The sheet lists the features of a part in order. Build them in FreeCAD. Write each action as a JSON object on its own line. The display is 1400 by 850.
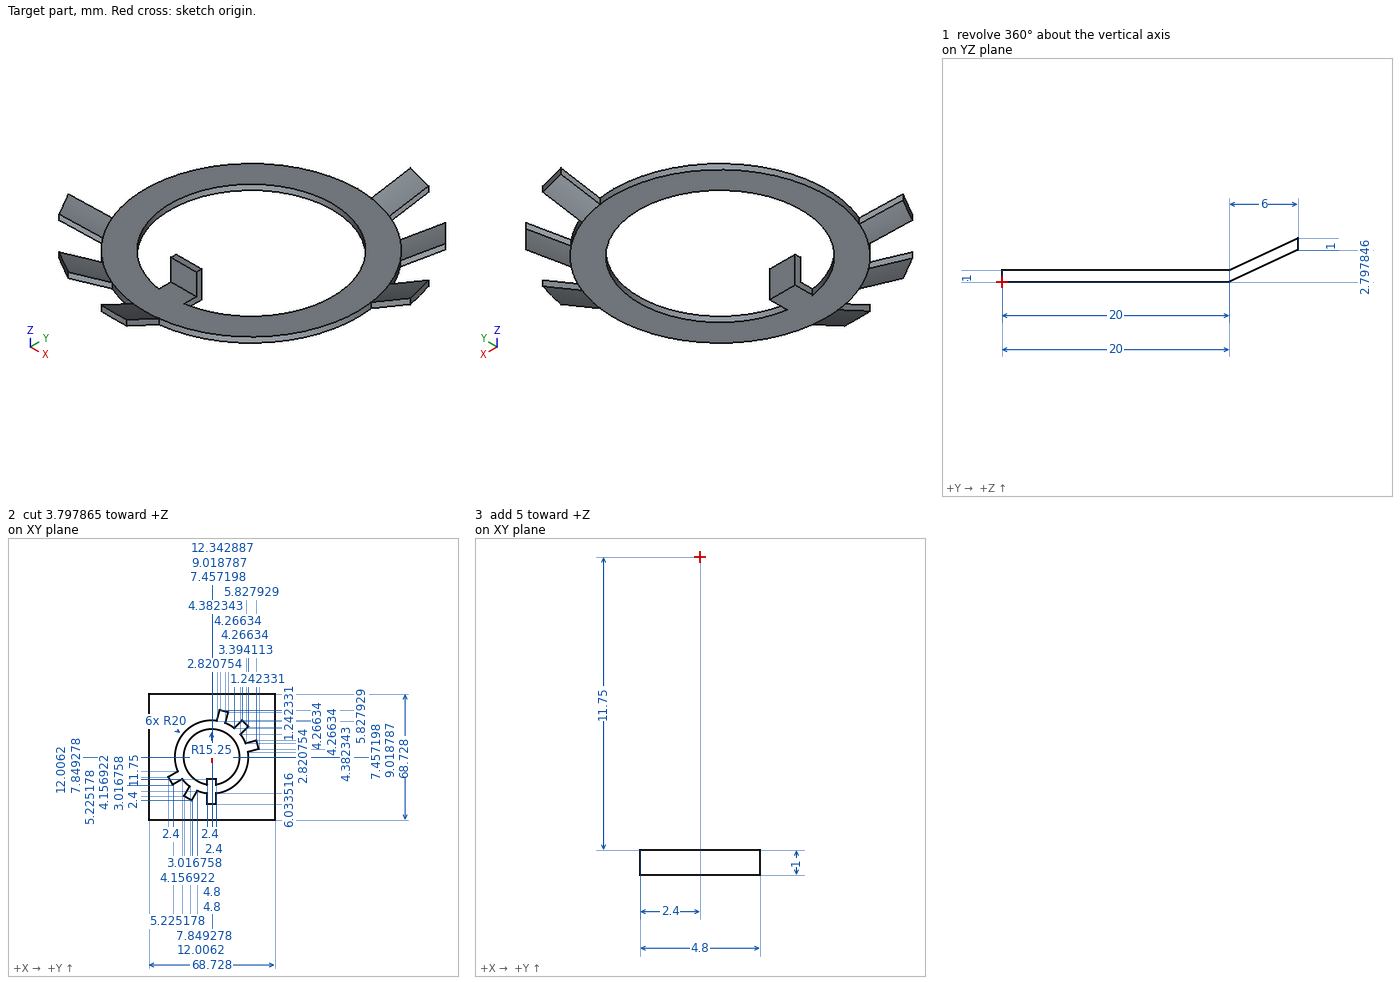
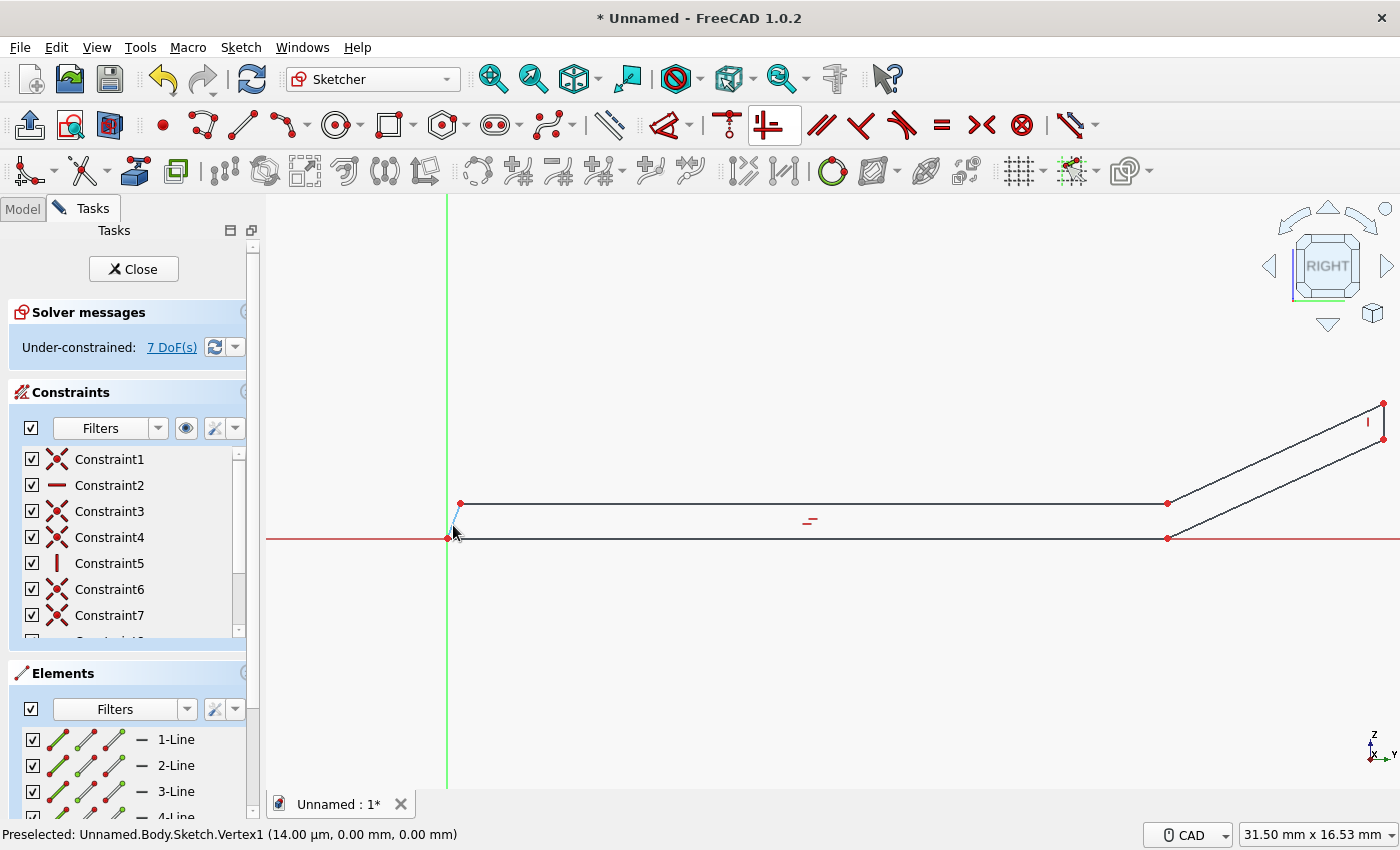
{"action": "left_click", "coordinate": [453, 525]}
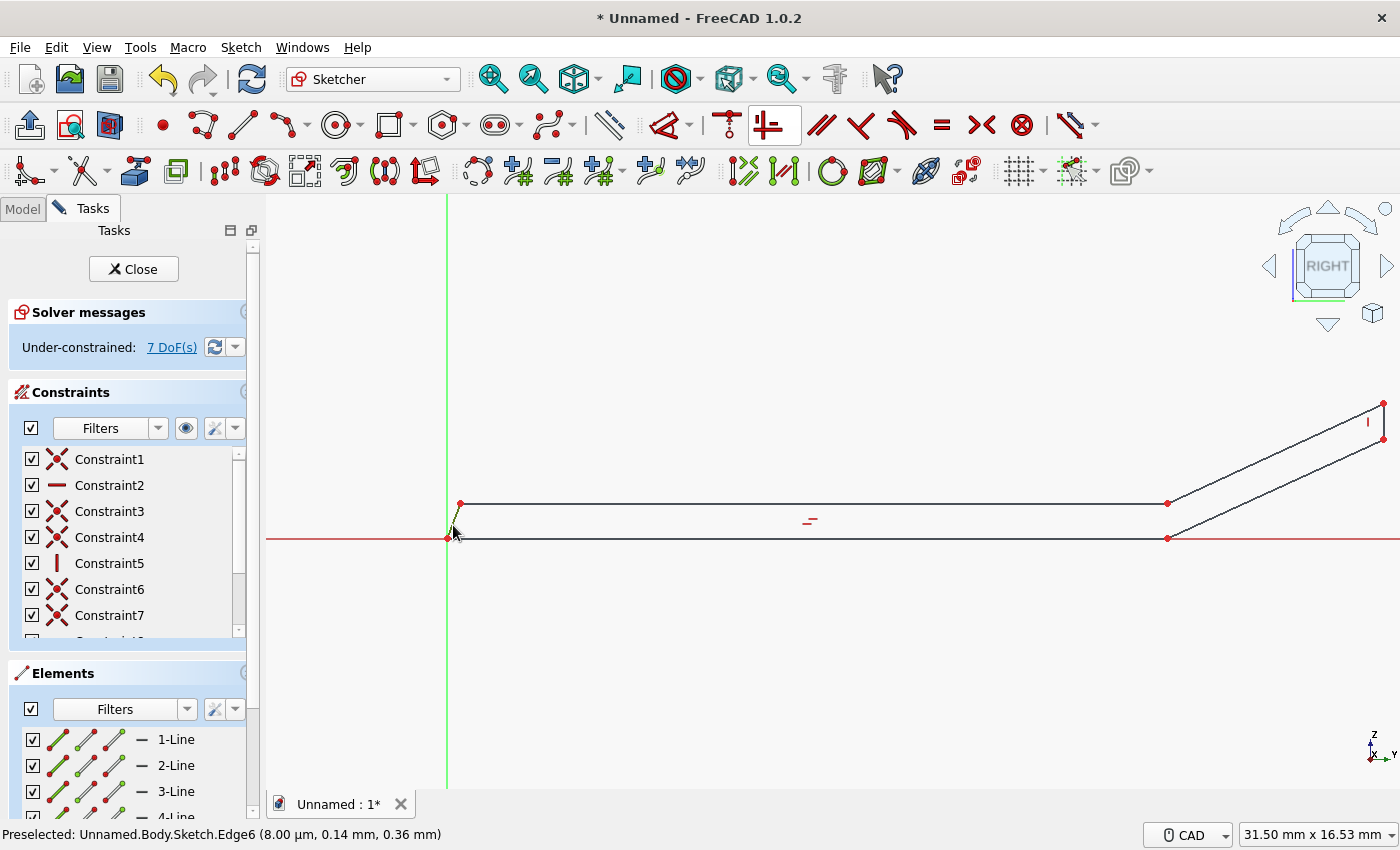
{"action": "left_click", "coordinate": [796, 126]}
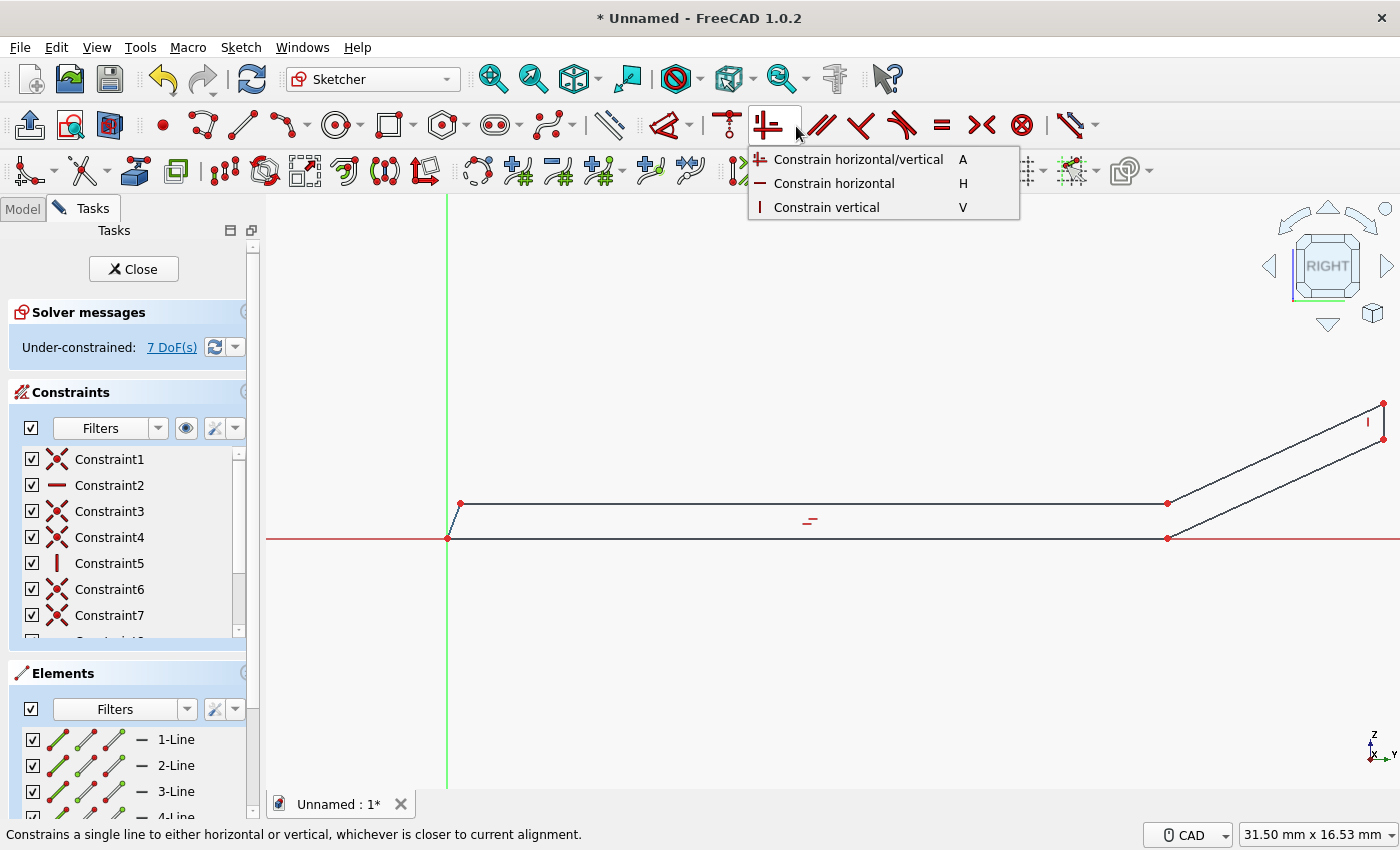
{"action": "left_click", "coordinate": [884, 207]}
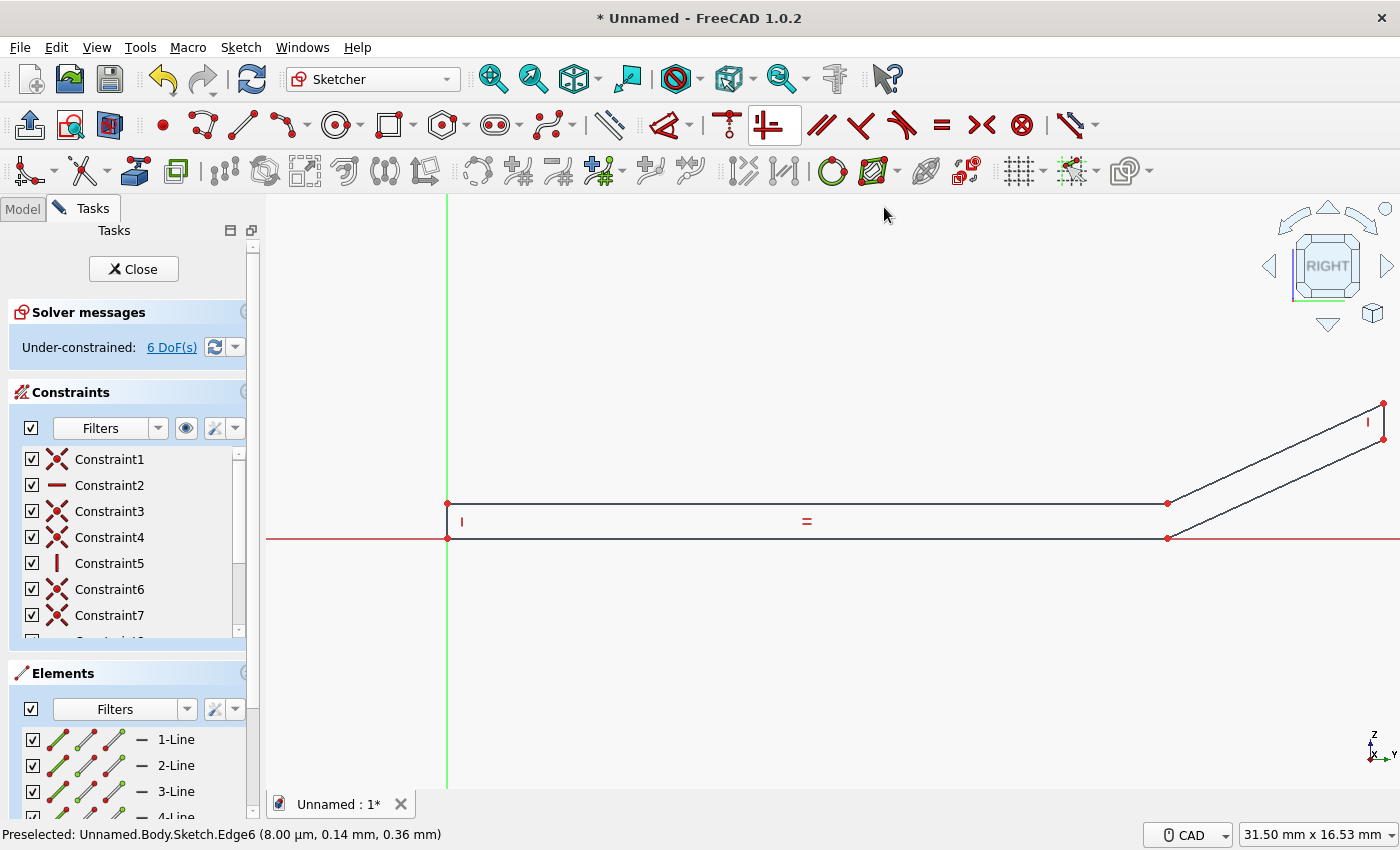
{"action": "left_click", "coordinate": [664, 126]}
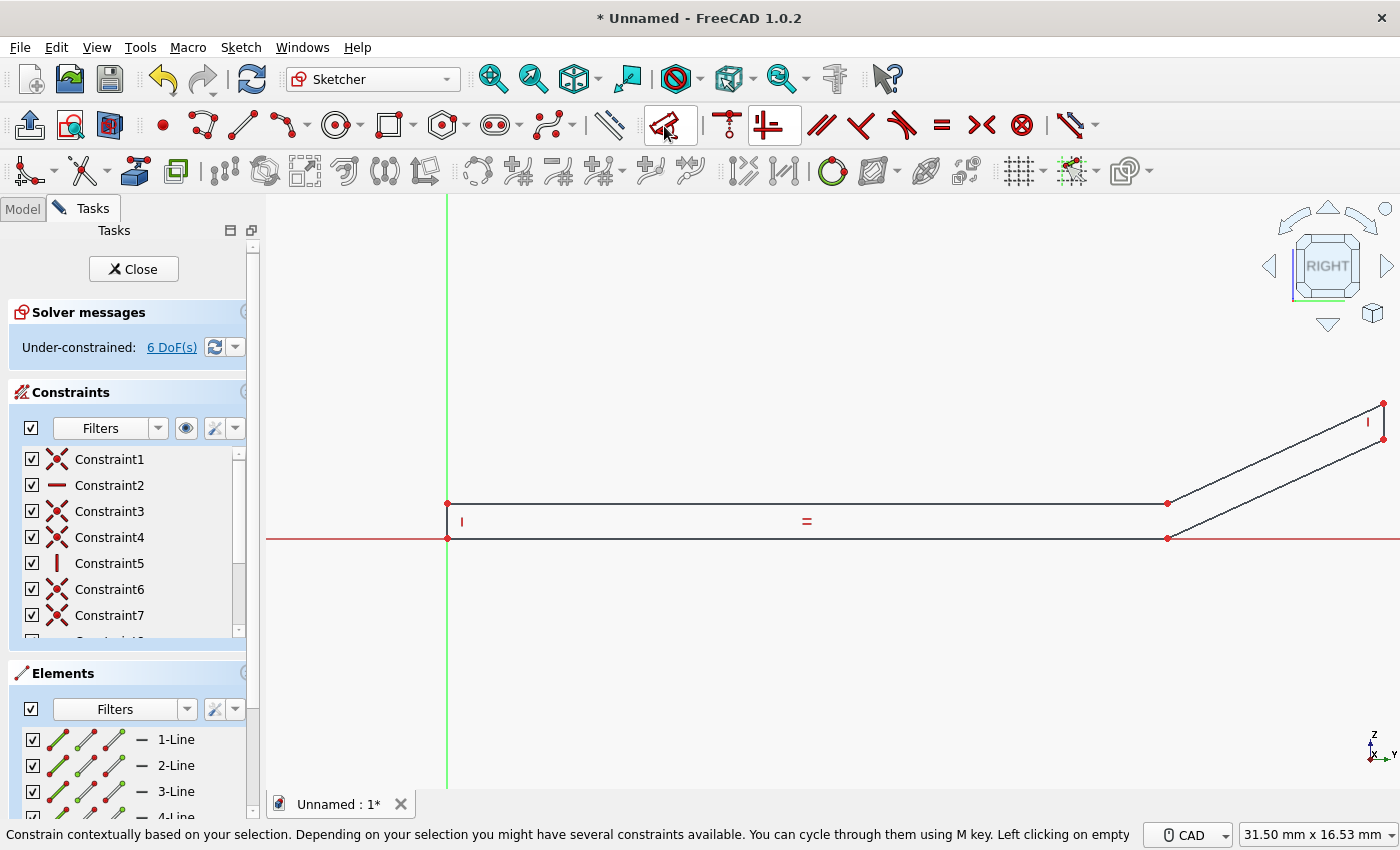
{"action": "scroll", "coordinate": [458, 535], "scroll_direction": "down", "scroll_amount": 2}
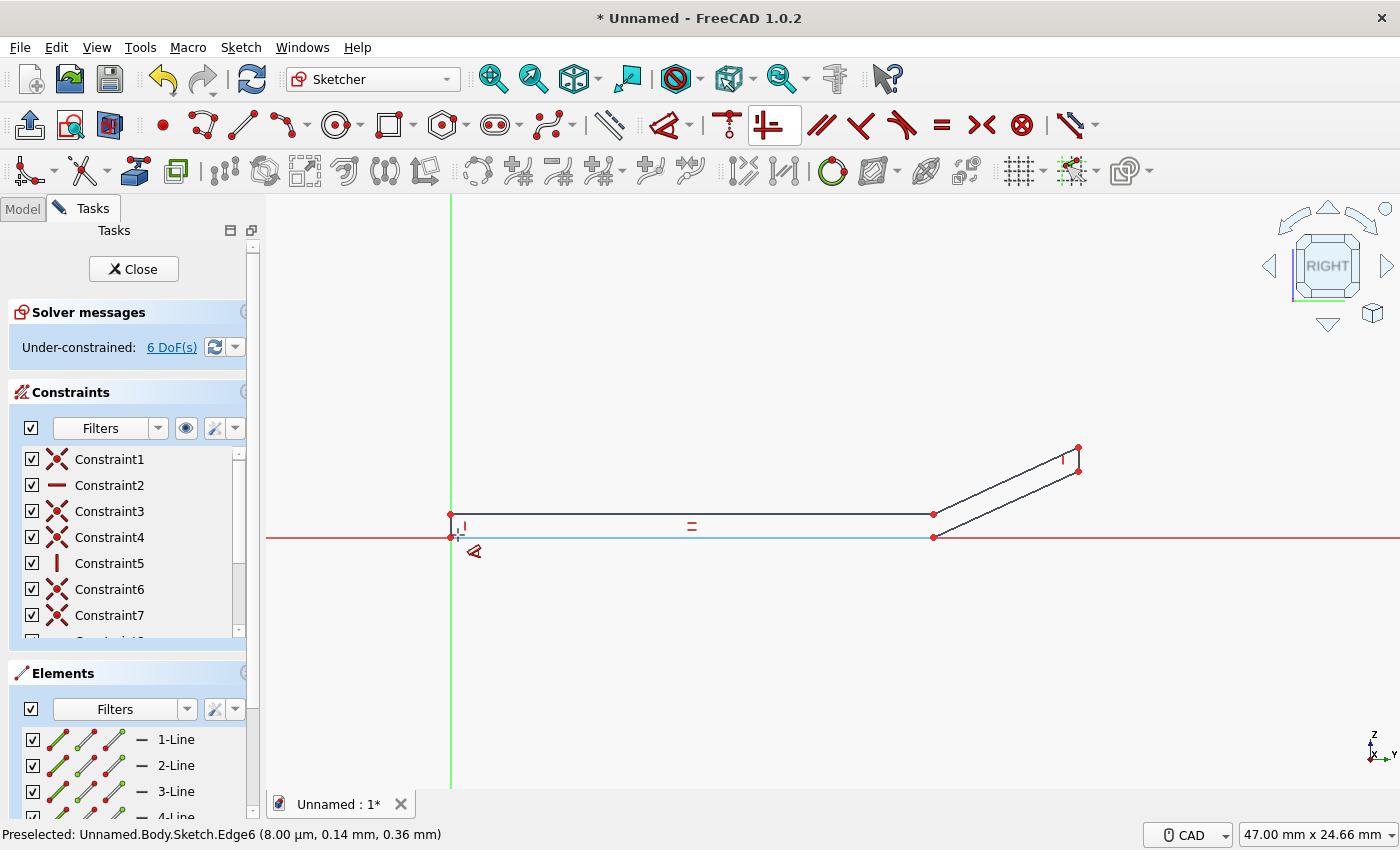
{"action": "scroll", "coordinate": [1079, 464], "scroll_direction": "up", "scroll_amount": 4}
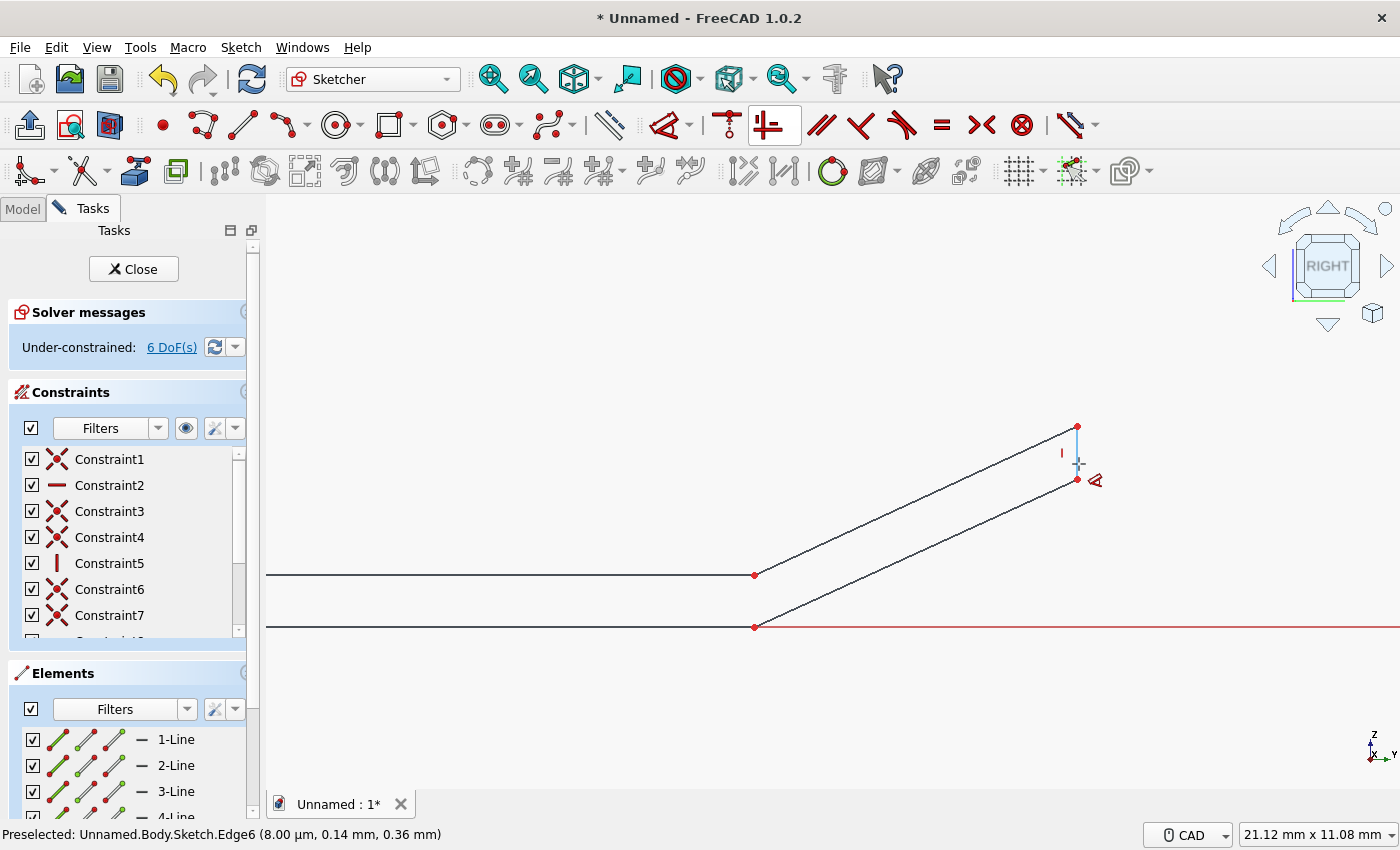
{"action": "left_click", "coordinate": [1077, 464]}
{"action": "left_click", "coordinate": [1111, 453]}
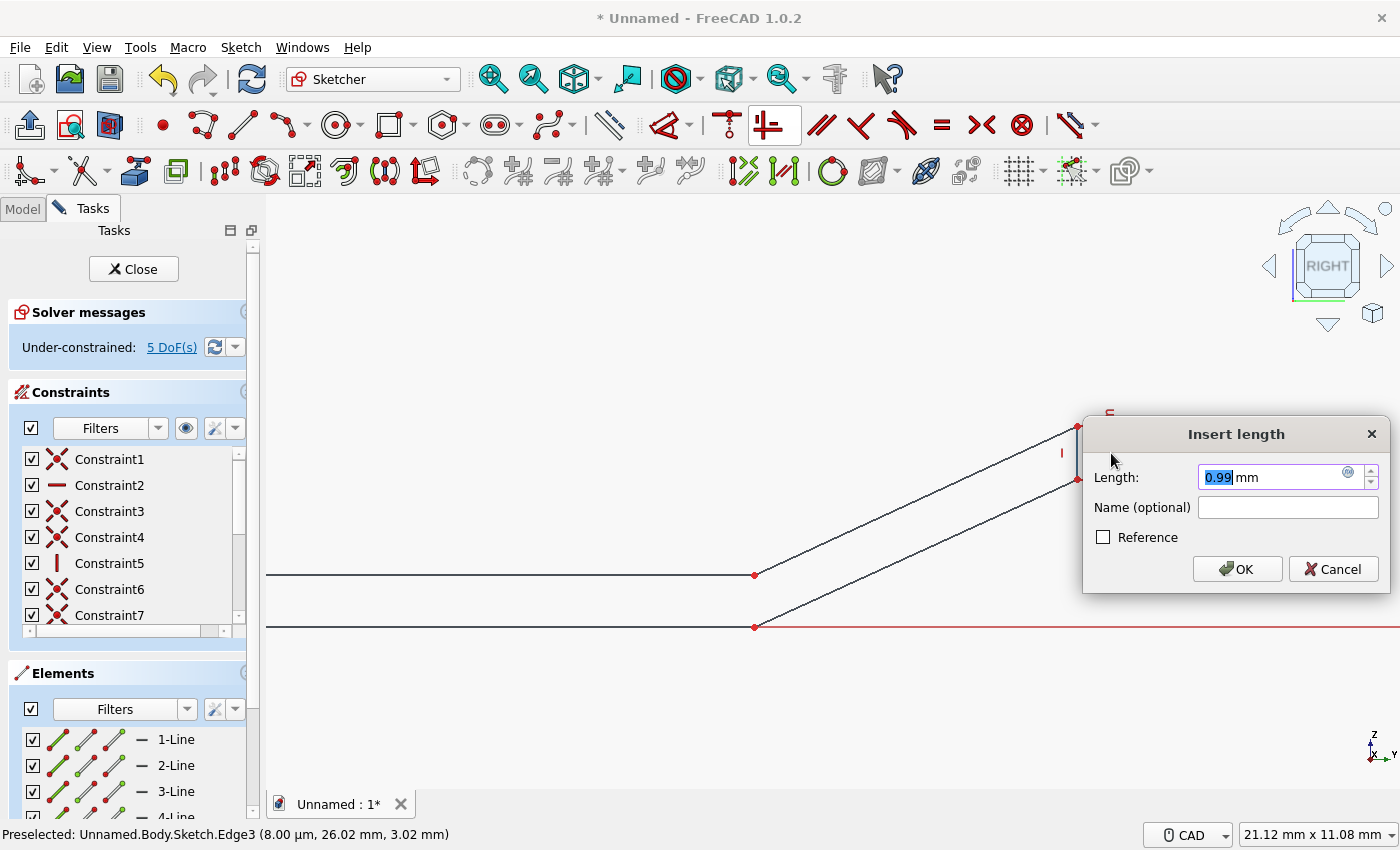
{"action": "type", "text": "1"}
{"action": "key", "text": "Return"}